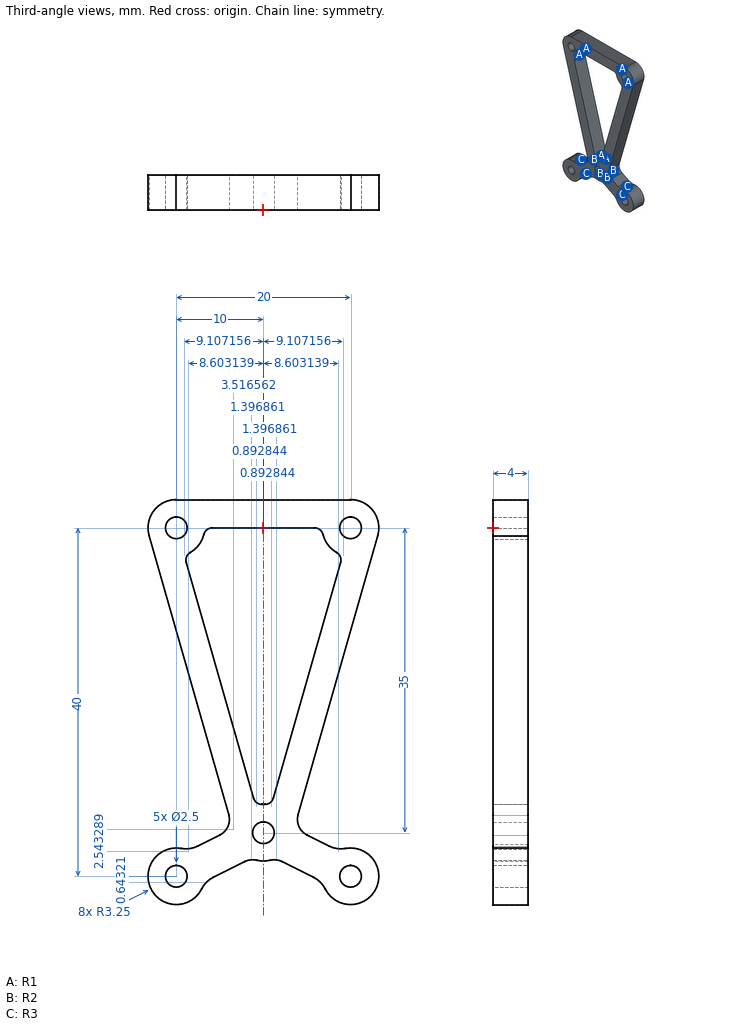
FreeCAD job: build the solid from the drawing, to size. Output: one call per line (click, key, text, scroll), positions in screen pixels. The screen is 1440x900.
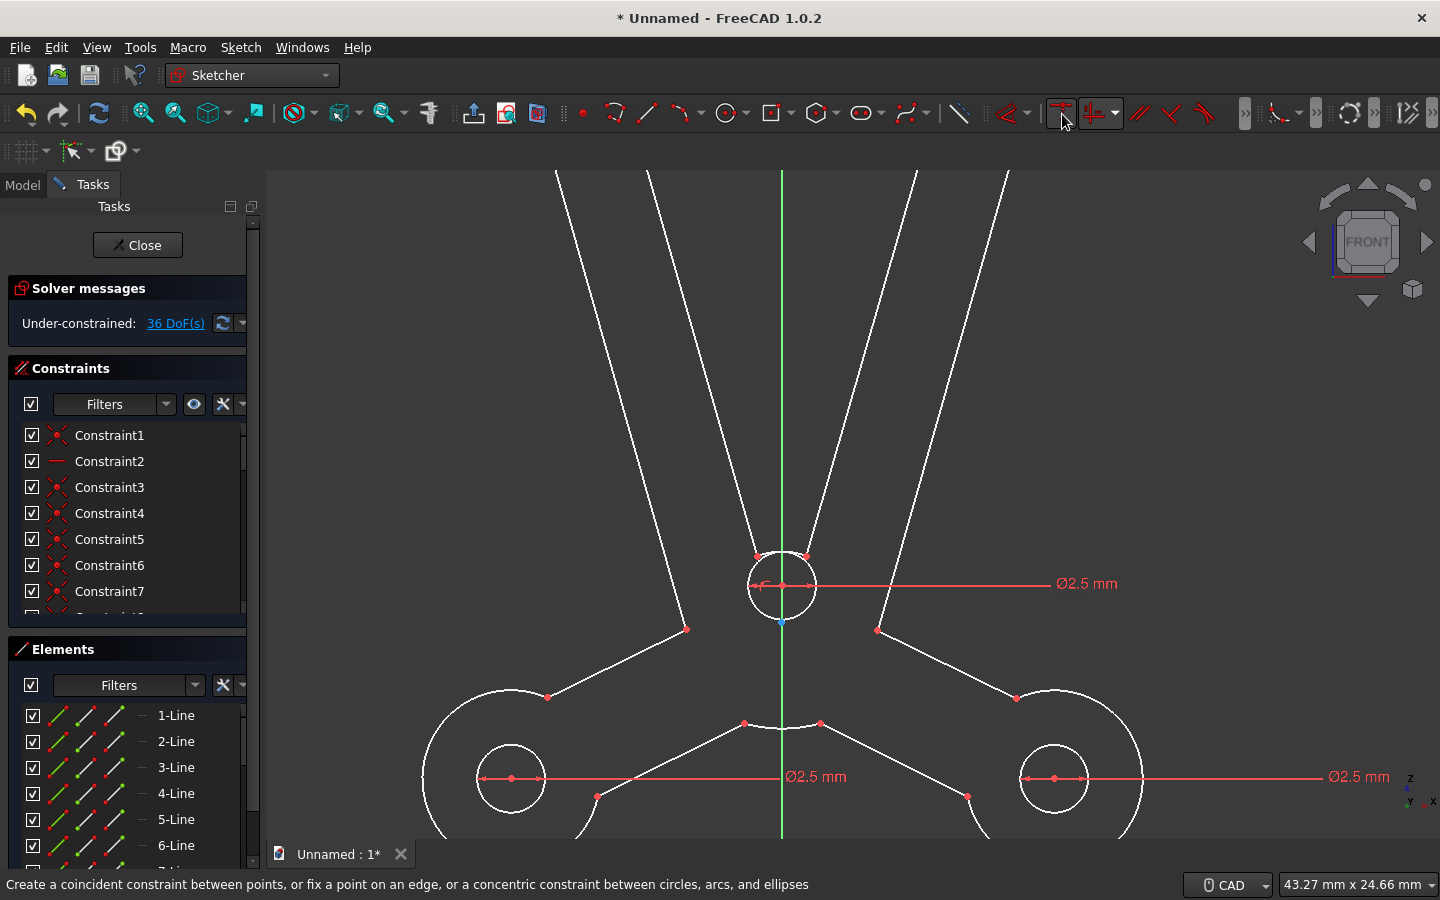
scroll(786, 677, down, 5)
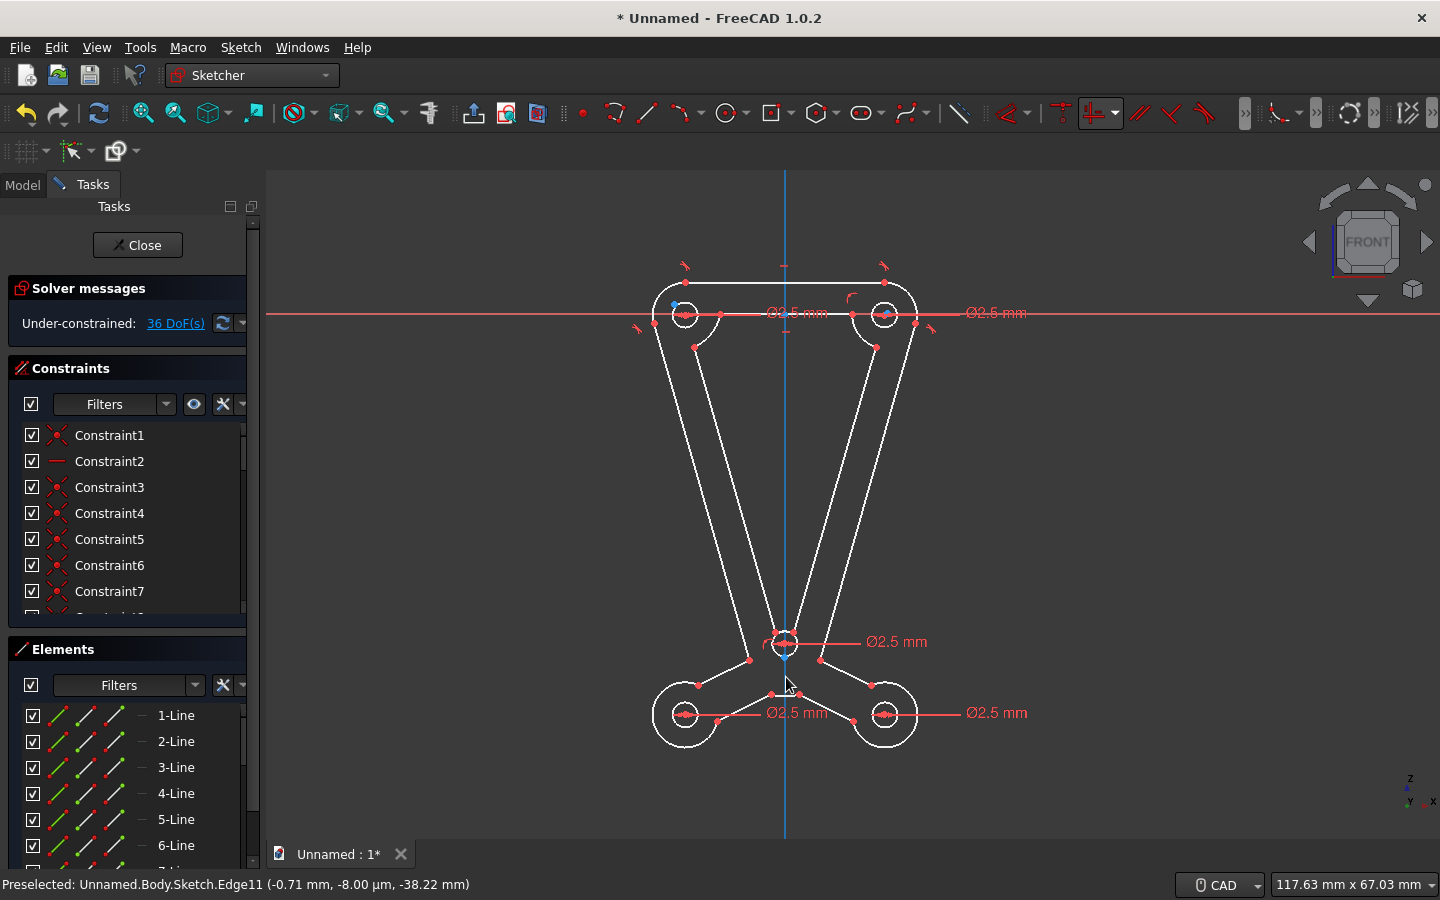
scroll(893, 306, up, 3)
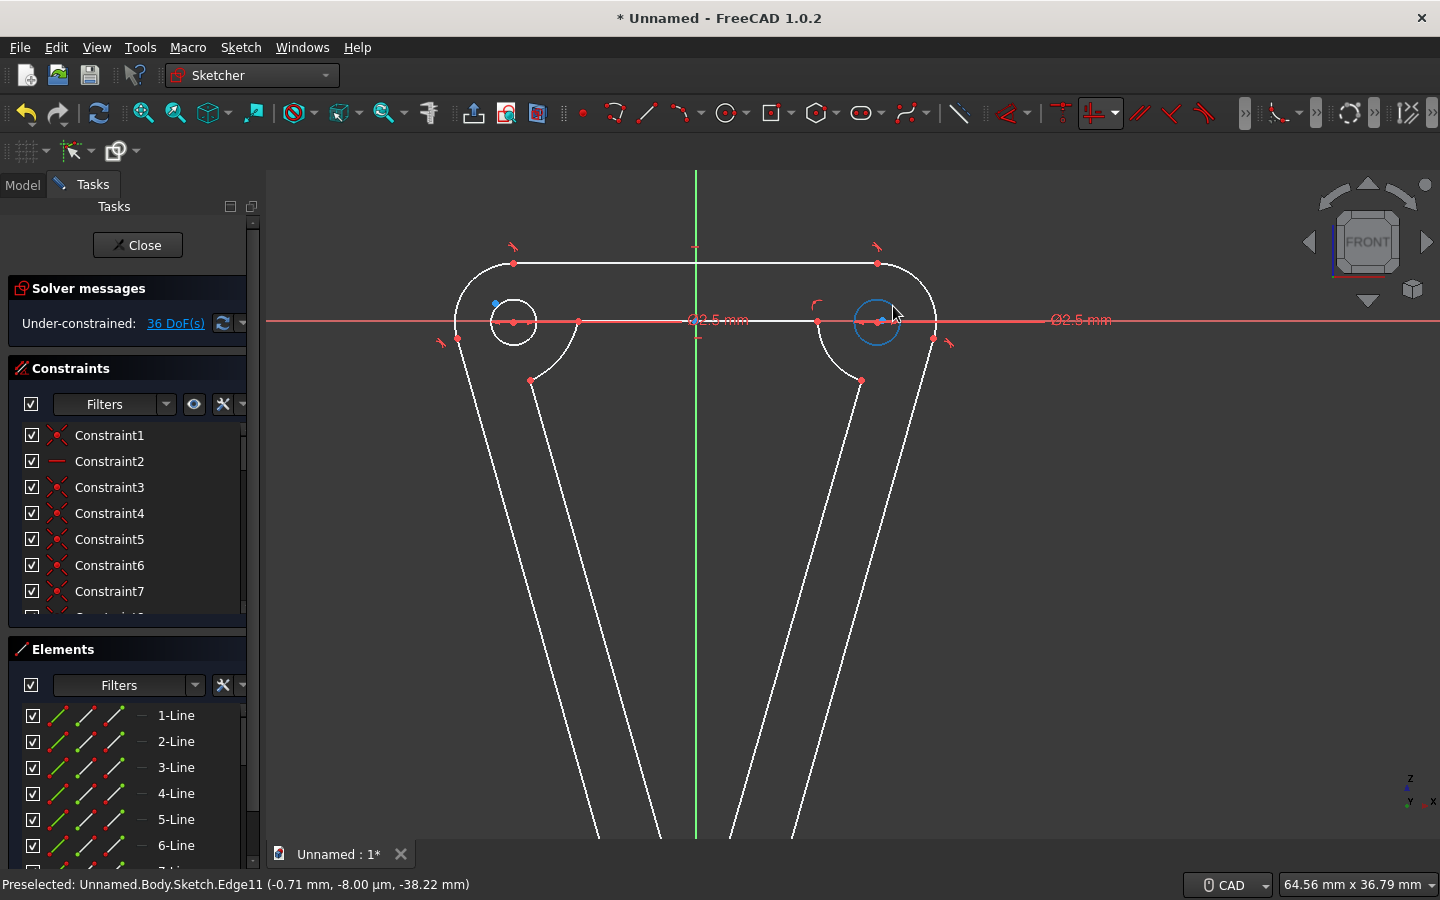
click(893, 306)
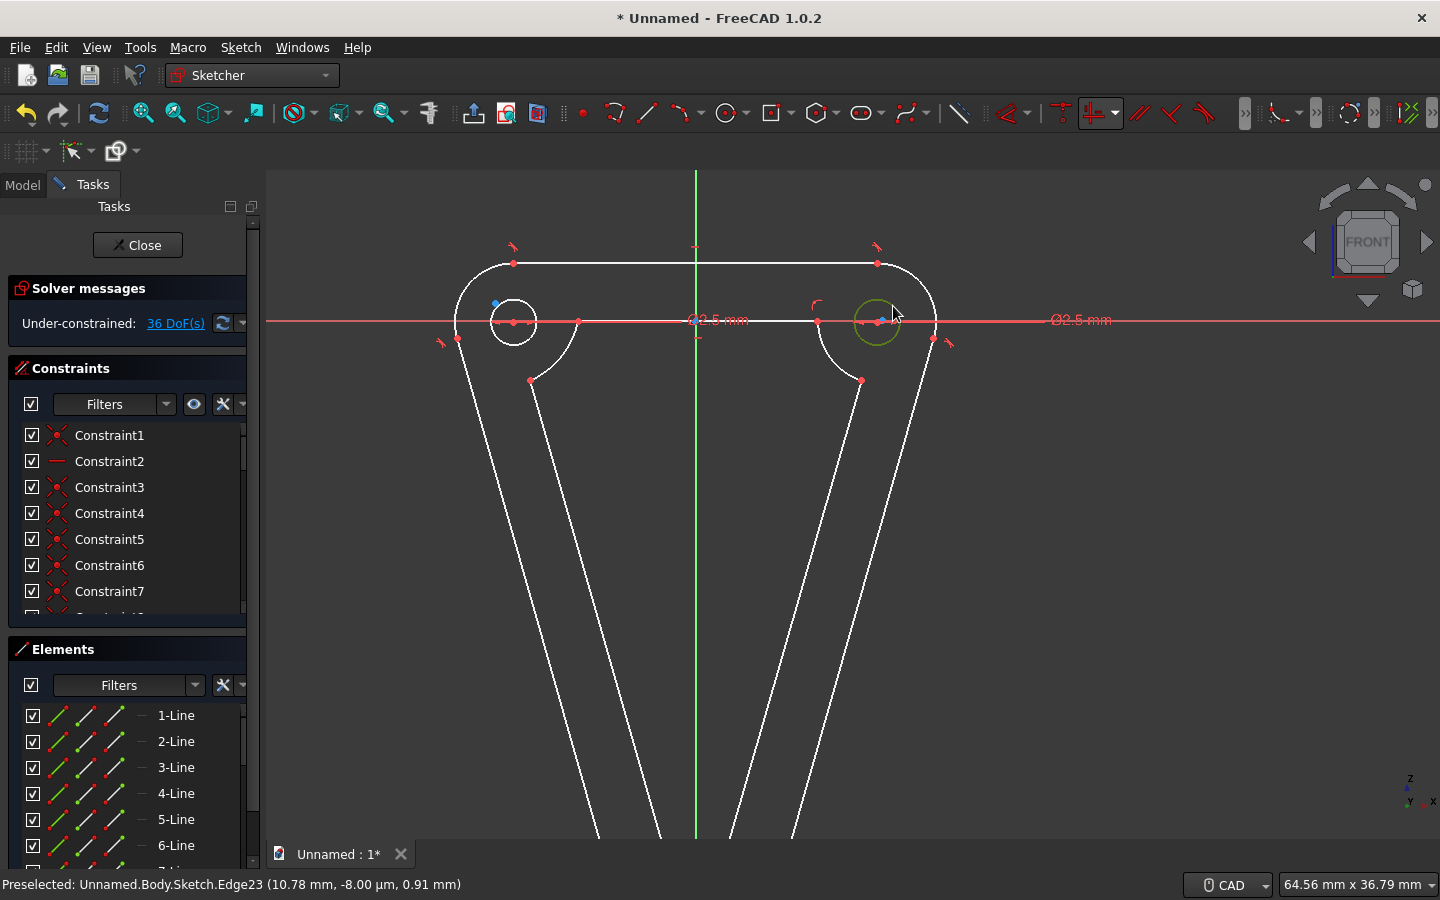
click(823, 344)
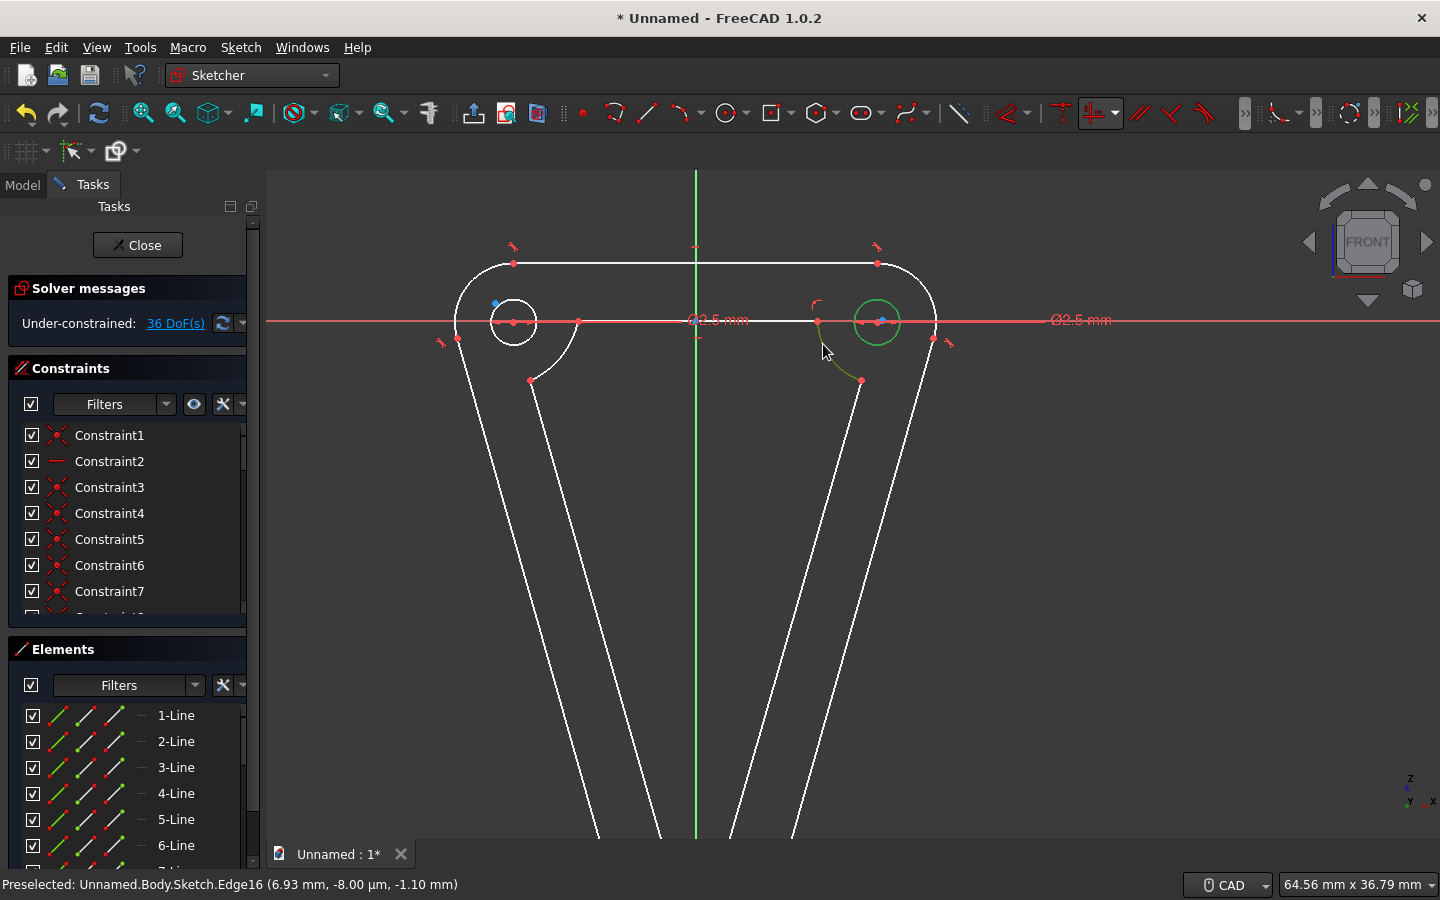
click(1062, 114)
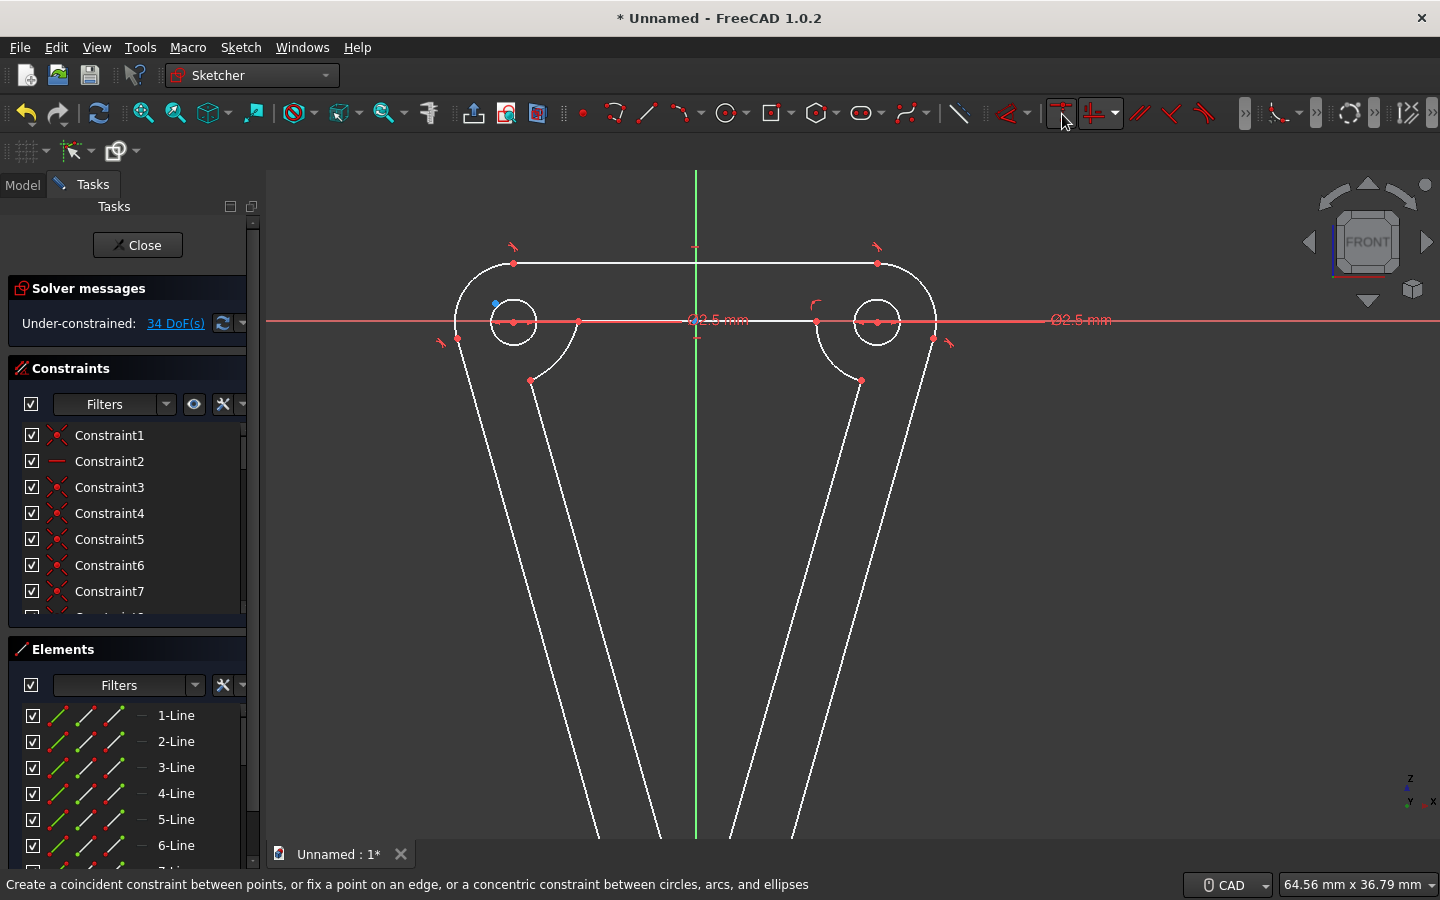
click(530, 306)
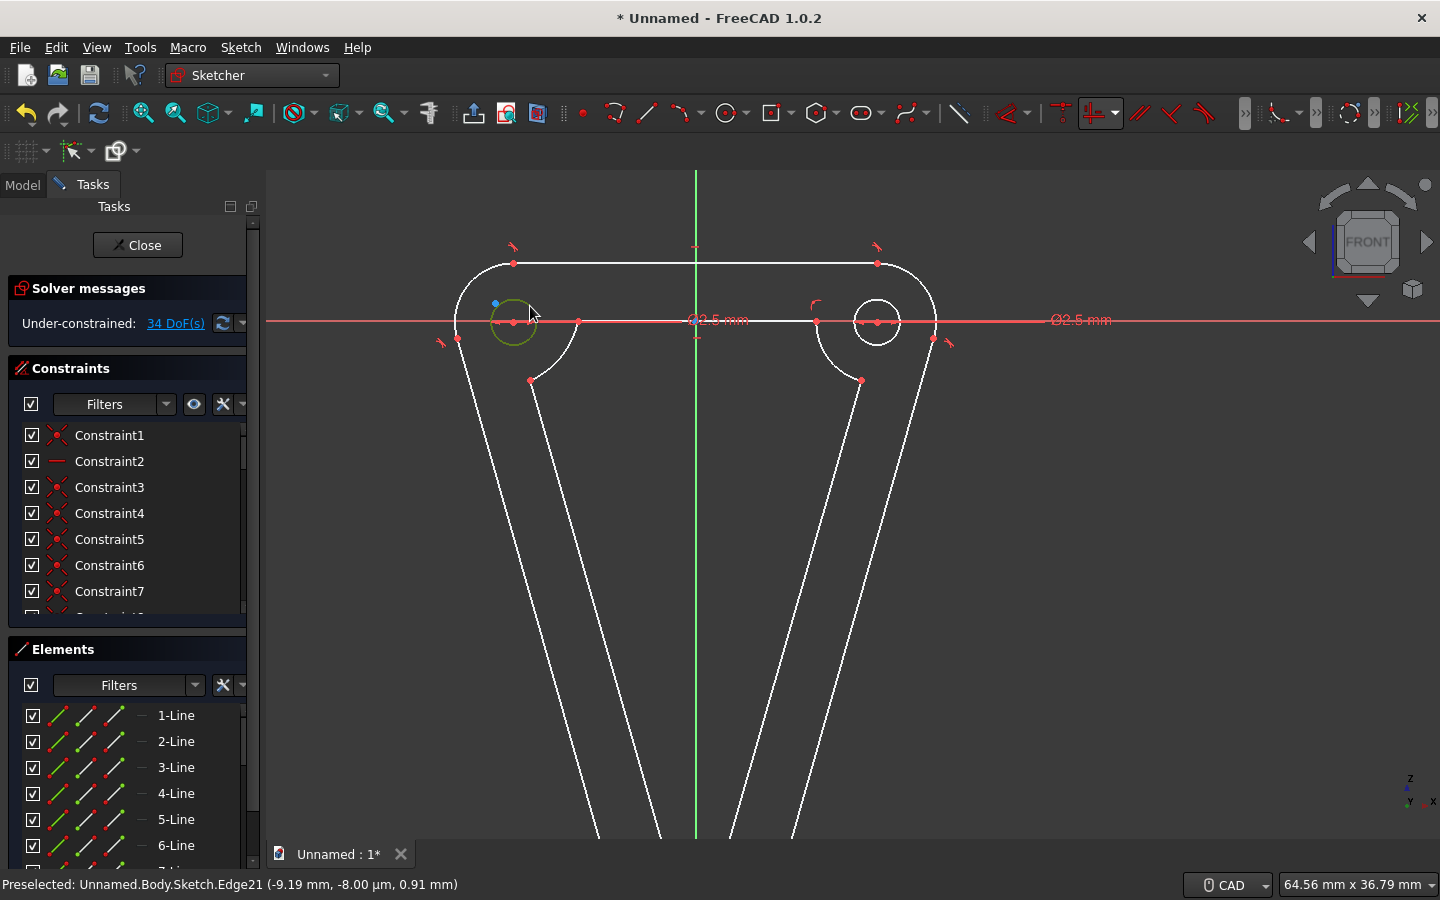
click(550, 368)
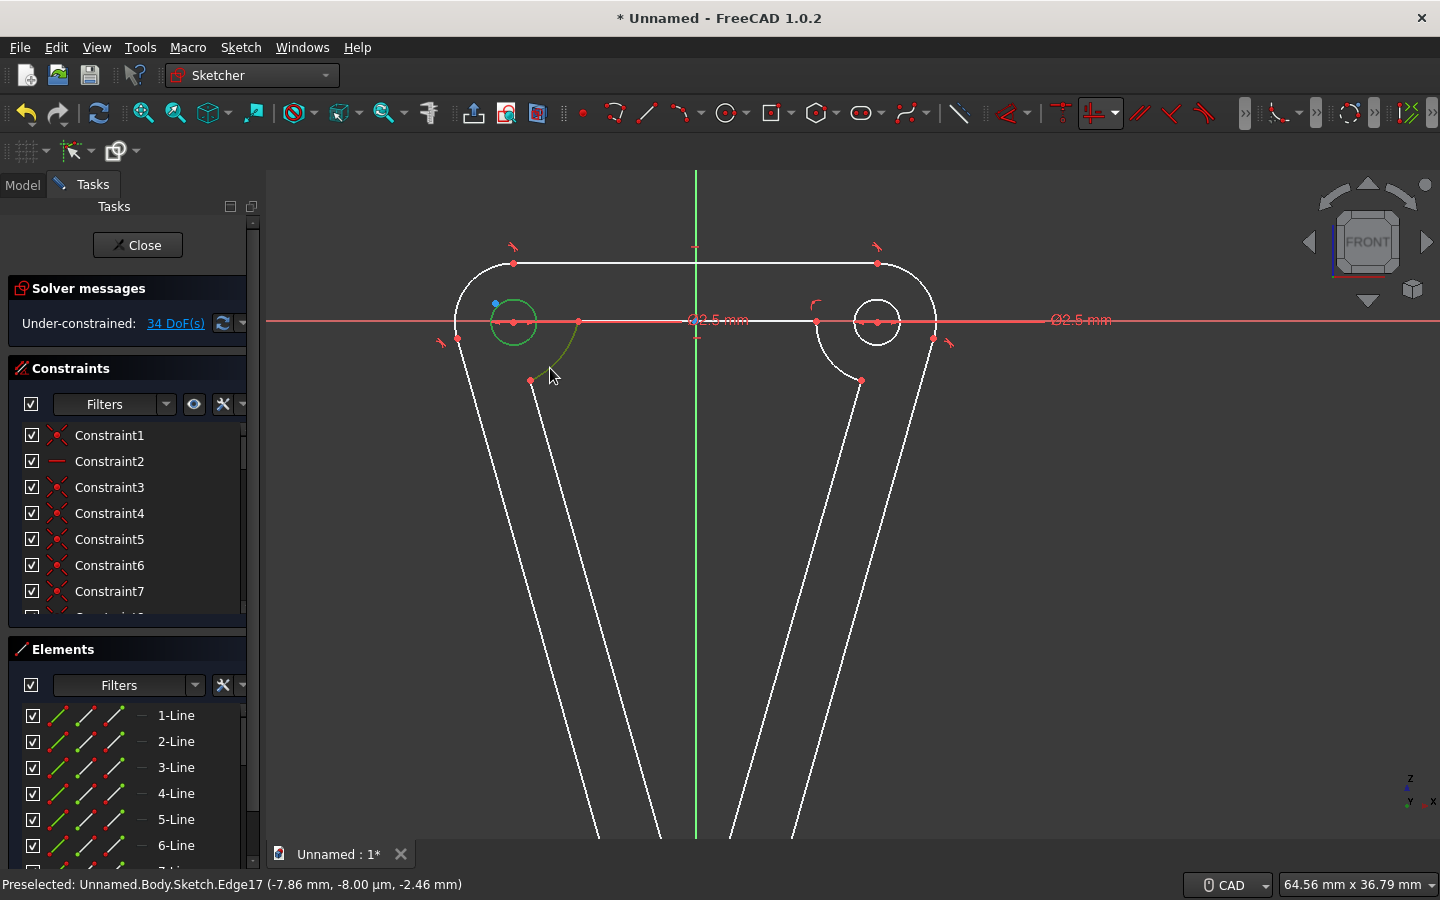
click(1062, 114)